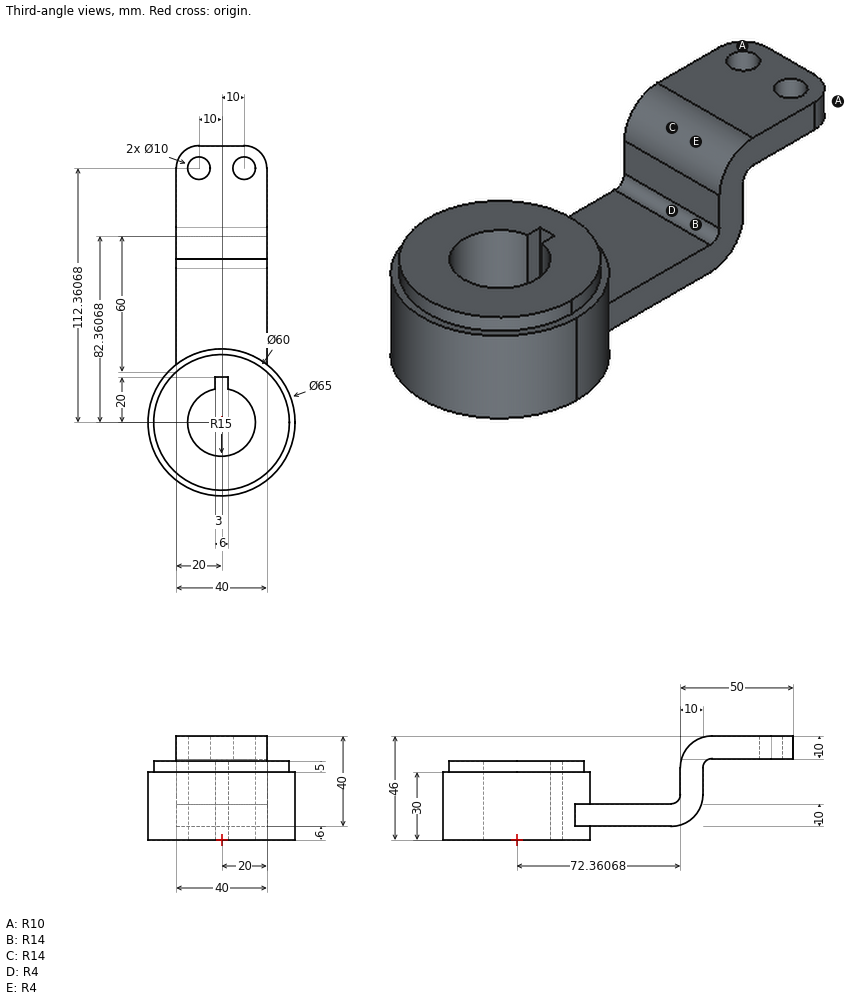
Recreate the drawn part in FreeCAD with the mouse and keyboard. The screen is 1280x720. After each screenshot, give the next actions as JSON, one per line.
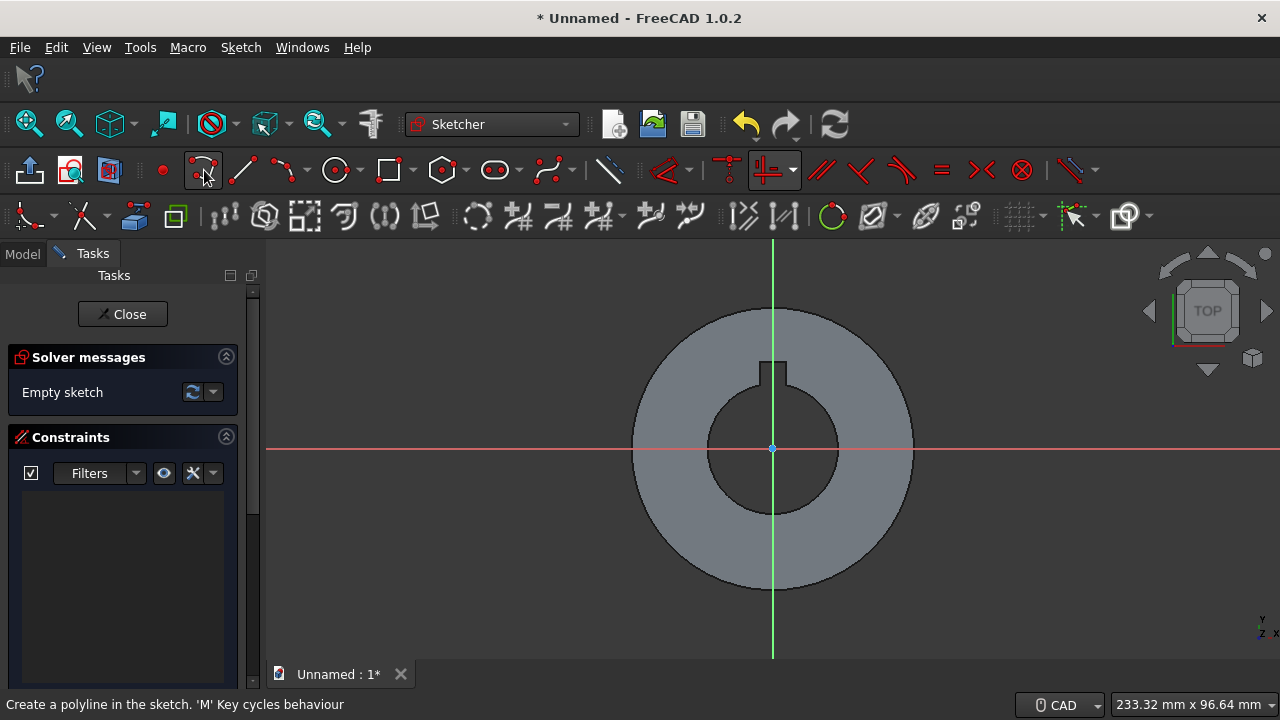
{"action": "left_click", "coordinate": [760, 385]}
{"action": "left_click", "coordinate": [760, 362]}
{"action": "left_click", "coordinate": [786, 362]}
{"action": "left_click", "coordinate": [786, 385]}
{"action": "right_click", "coordinate": [786, 385]}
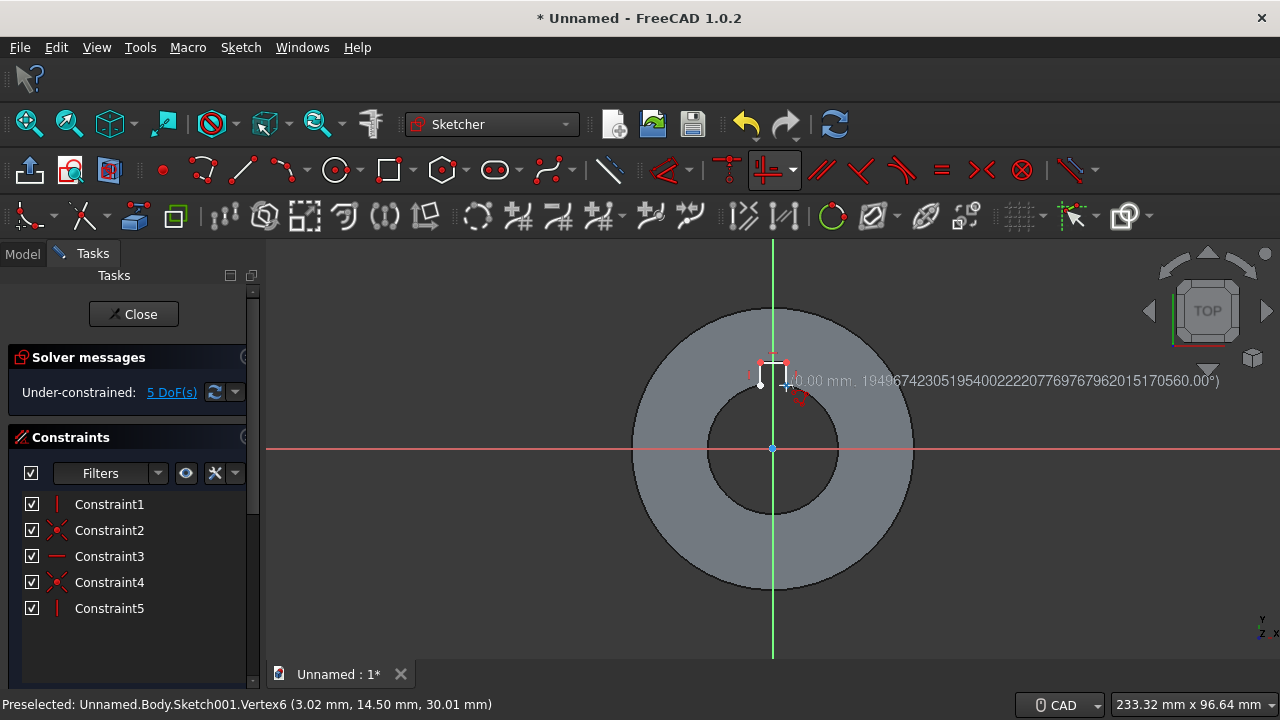
{"action": "key", "text": "g 3 a"}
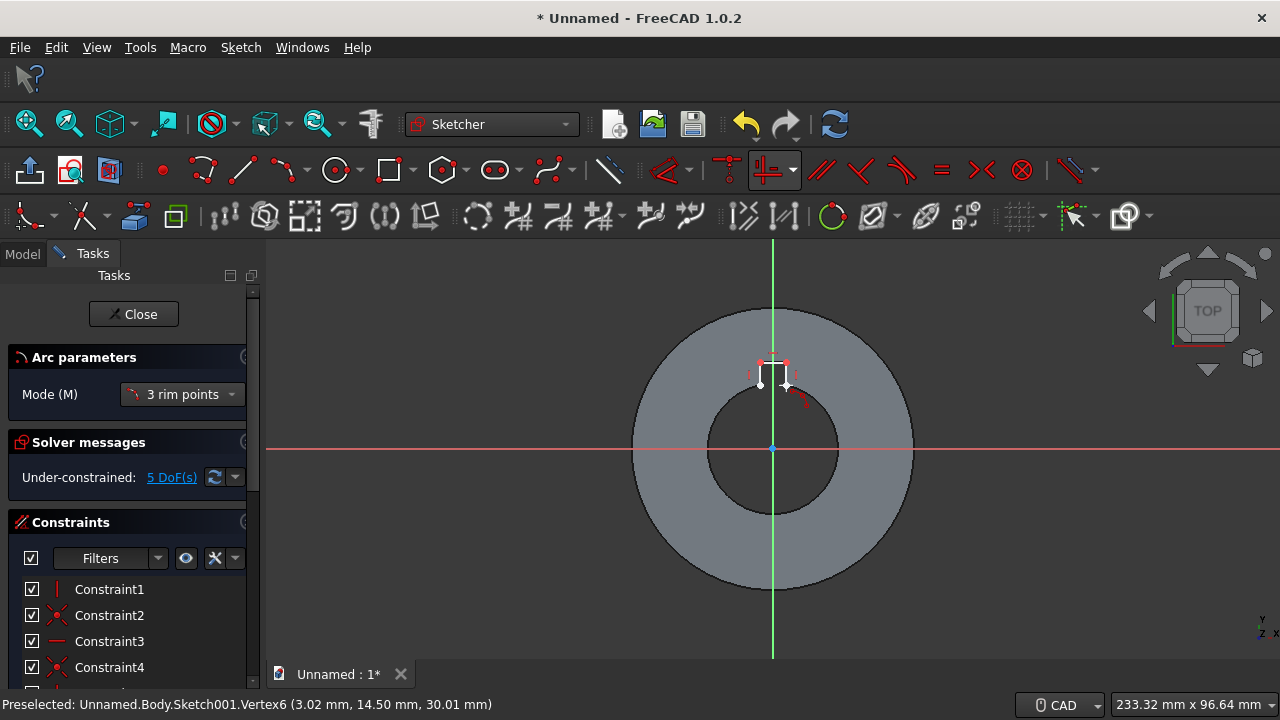
{"action": "scroll", "coordinate": [786, 385], "scroll_direction": "up", "scroll_amount": 2}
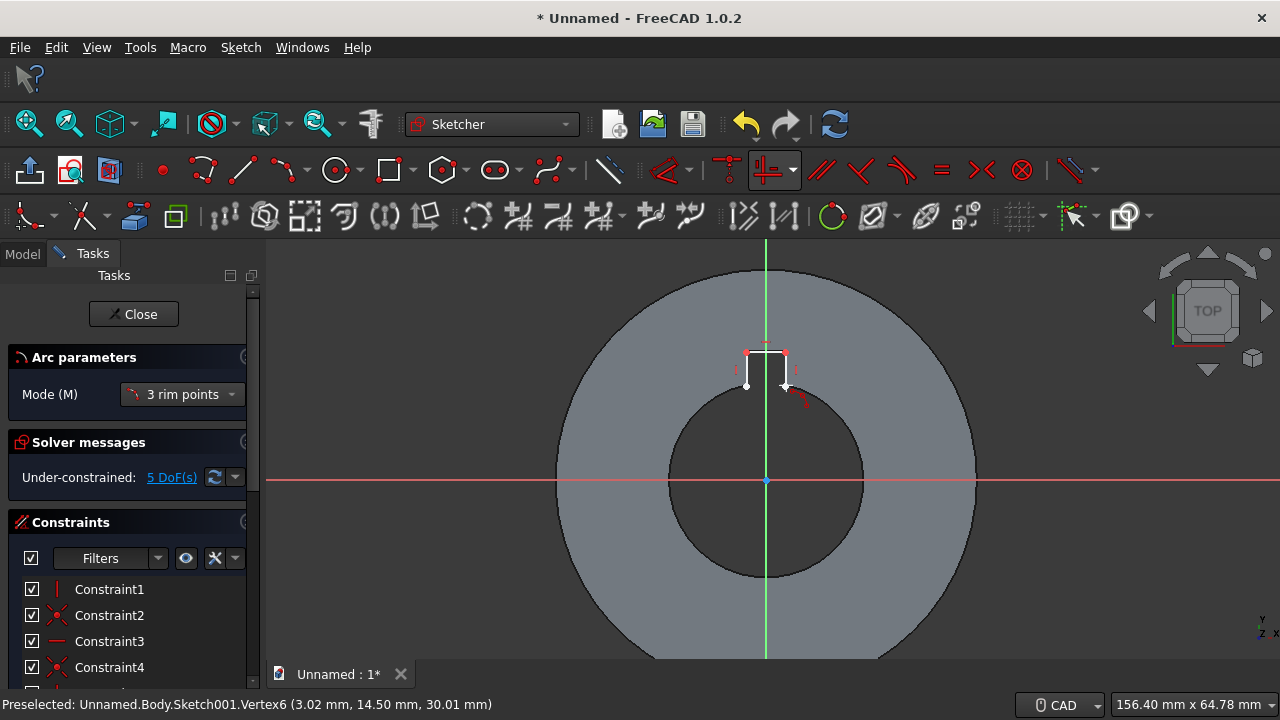
{"action": "left_click", "coordinate": [786, 386]}
{"action": "left_click", "coordinate": [747, 386]}
{"action": "left_click", "coordinate": [712, 561]}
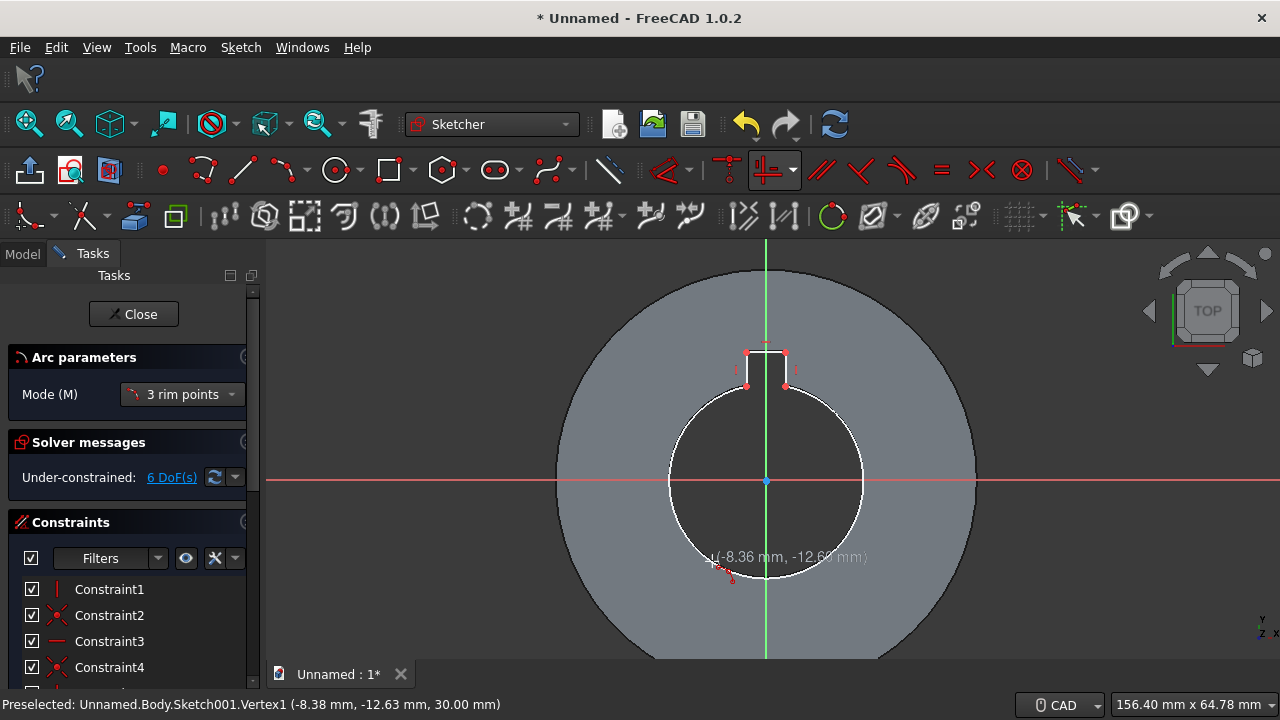
{"action": "key", "text": "g c"}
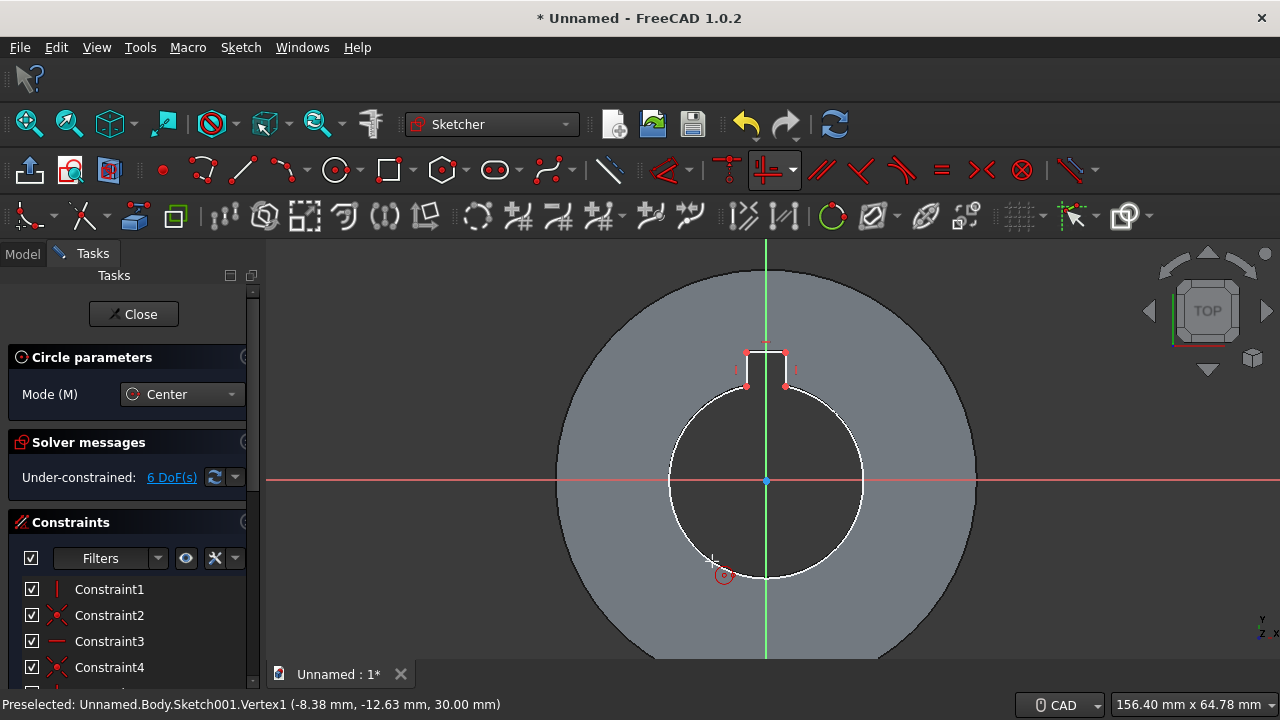
{"action": "left_click", "coordinate": [766, 480]}
{"action": "left_click", "coordinate": [904, 343]}
{"action": "key", "text": "Escape"}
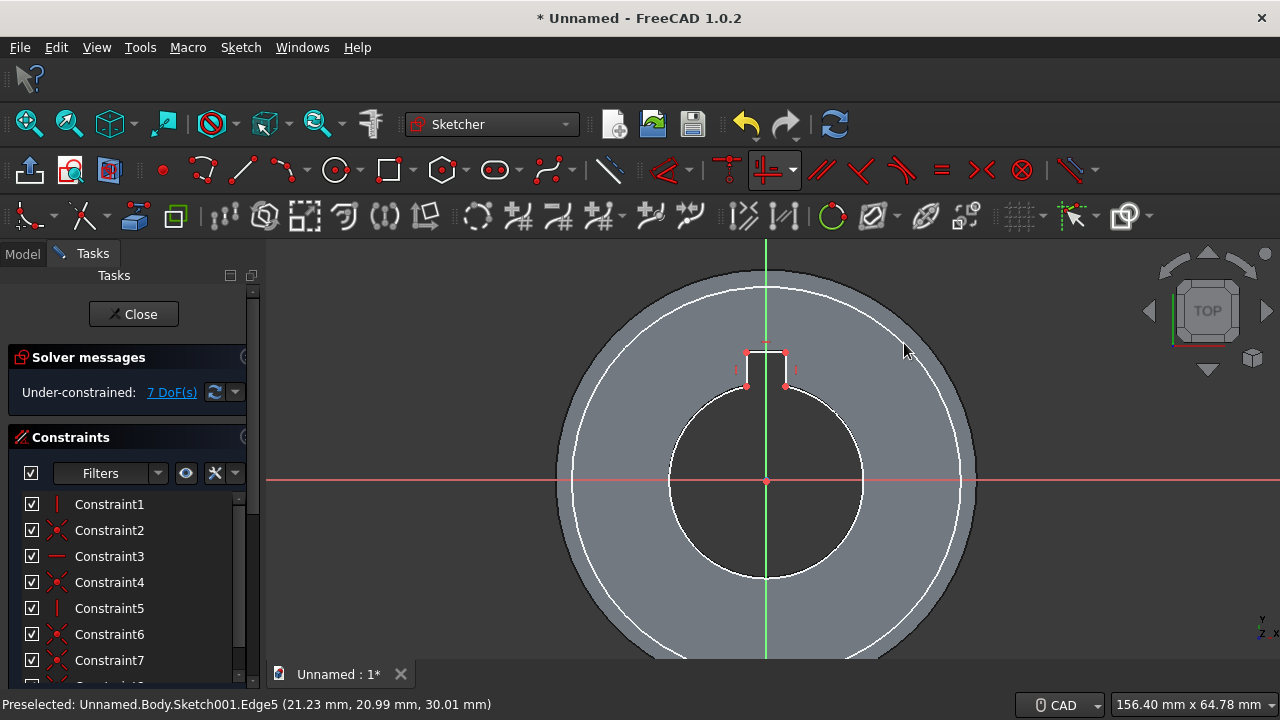
{"action": "left_click_drag", "start_coordinate": [756, 470], "coordinate": [776, 491]}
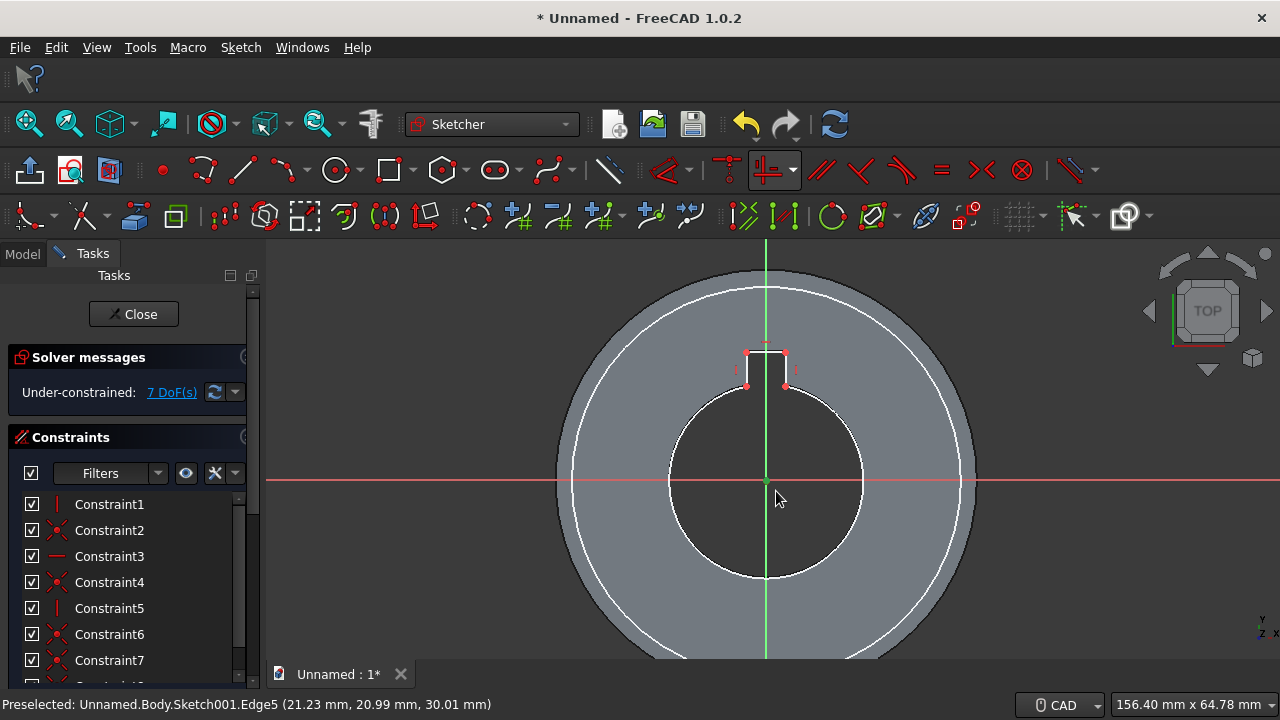
{"action": "key", "text": "c"}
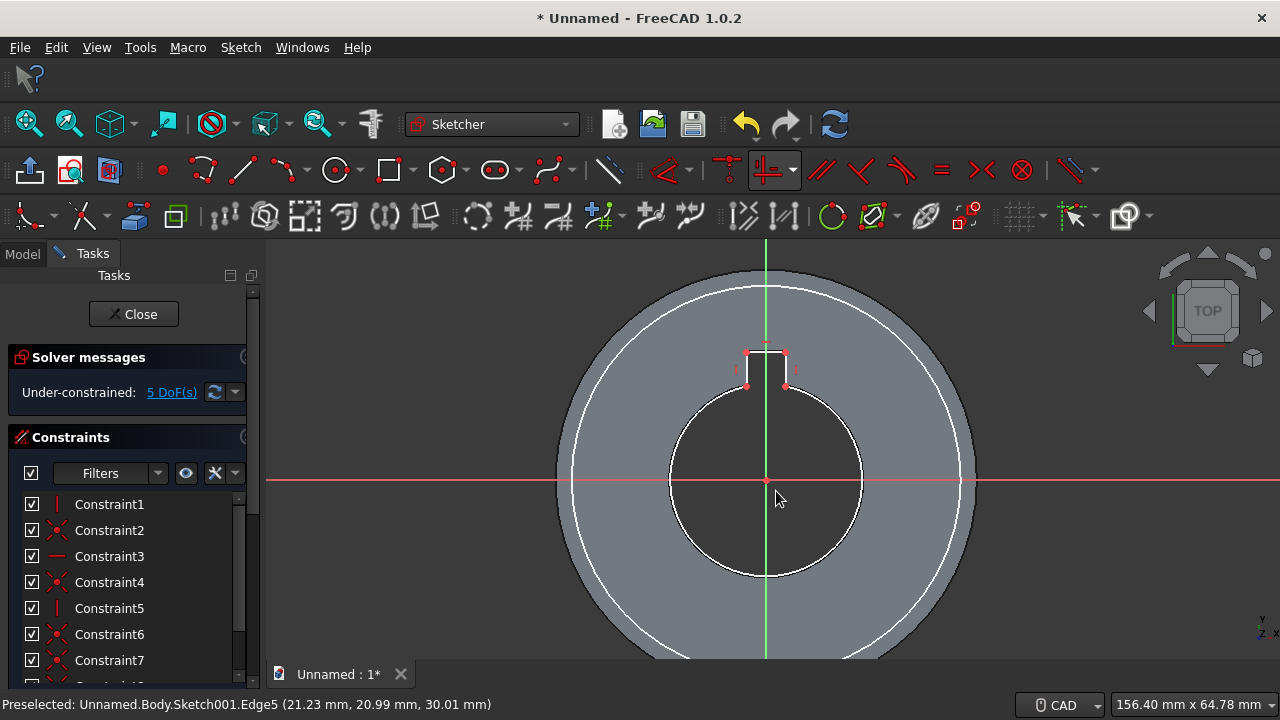
{"action": "key", "text": "d"}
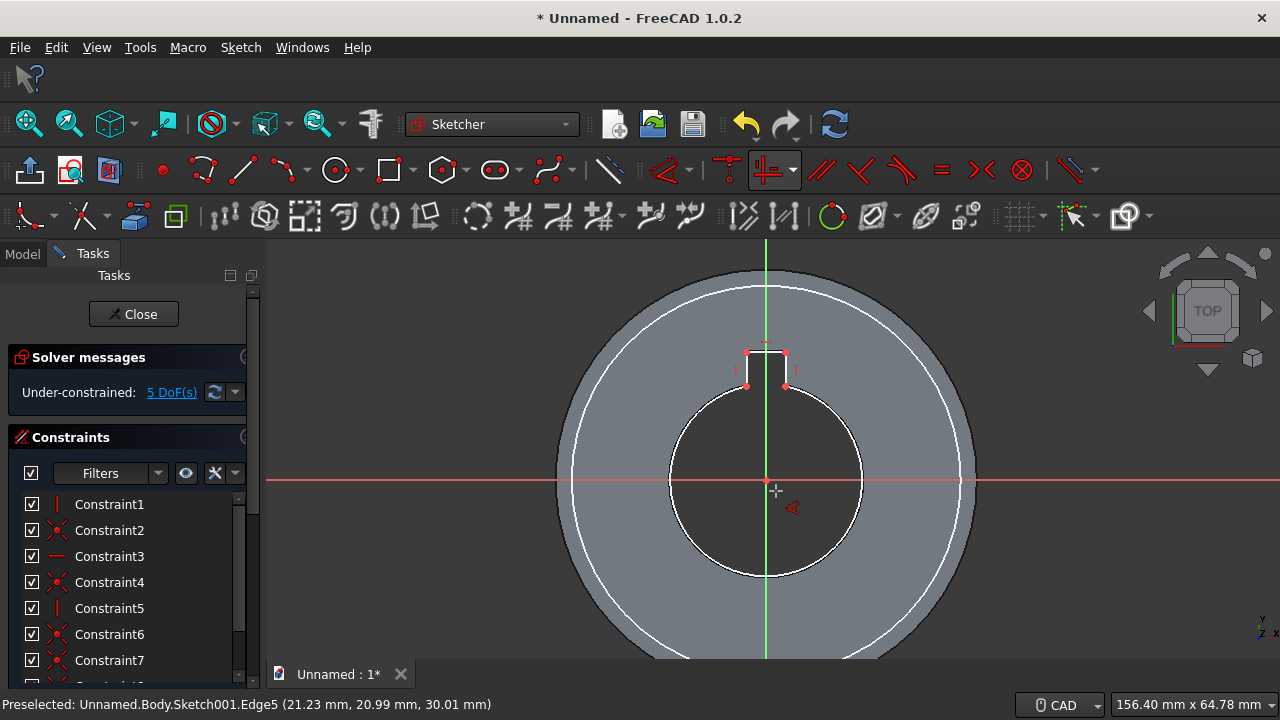
{"action": "left_click", "coordinate": [678, 517]}
{"action": "left_click", "coordinate": [648, 529]}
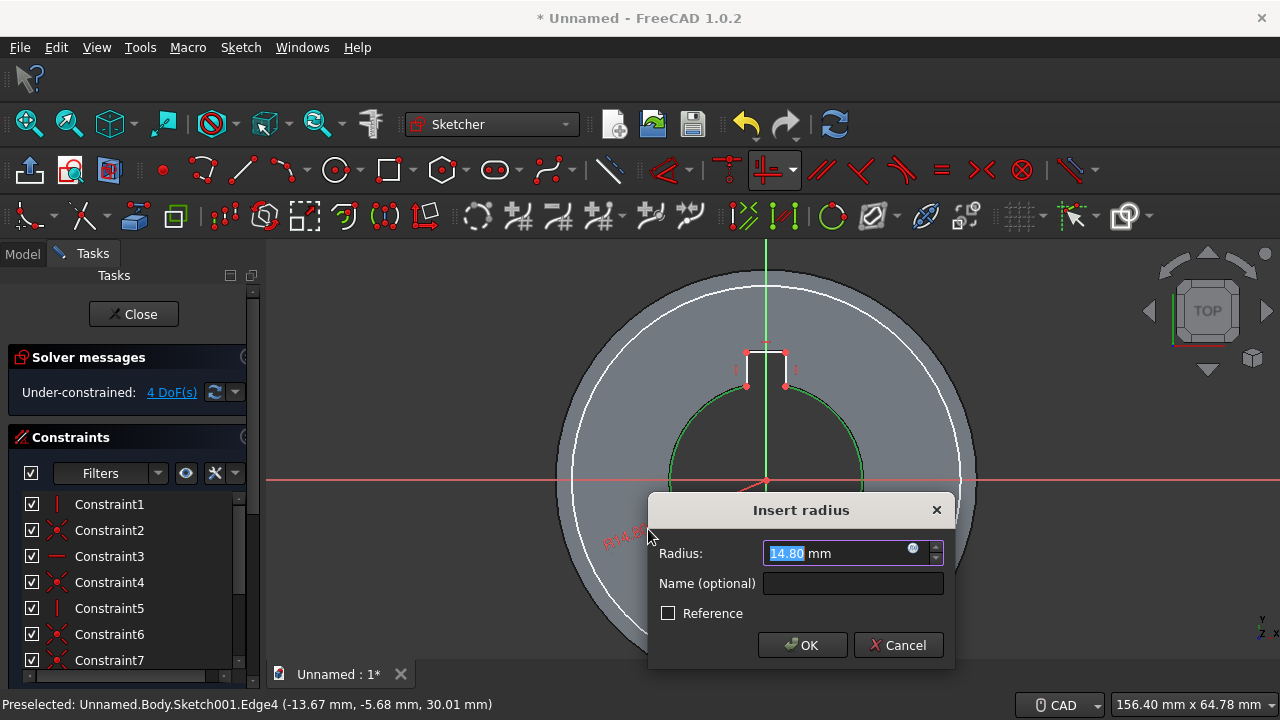
{"action": "type", "text": "15"}
{"action": "key", "text": "Return"}